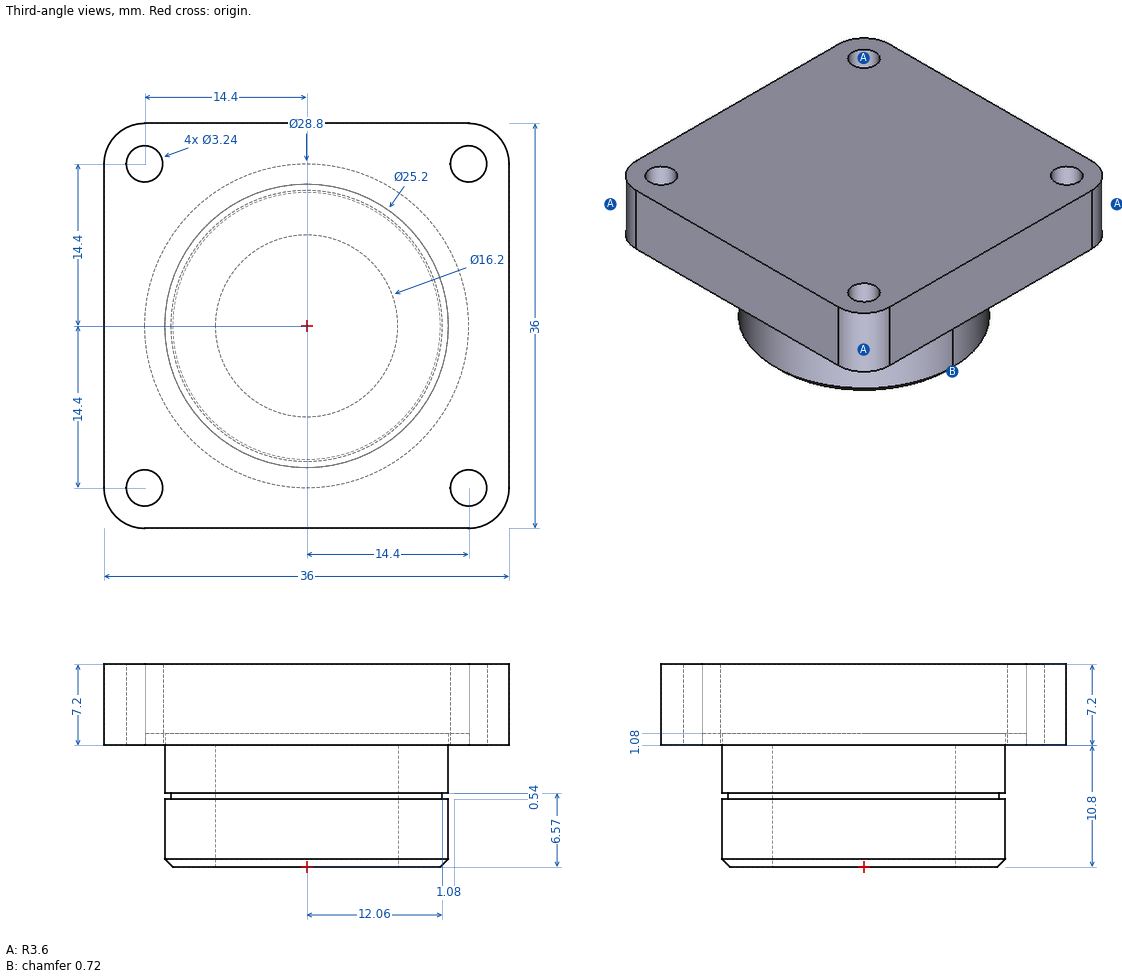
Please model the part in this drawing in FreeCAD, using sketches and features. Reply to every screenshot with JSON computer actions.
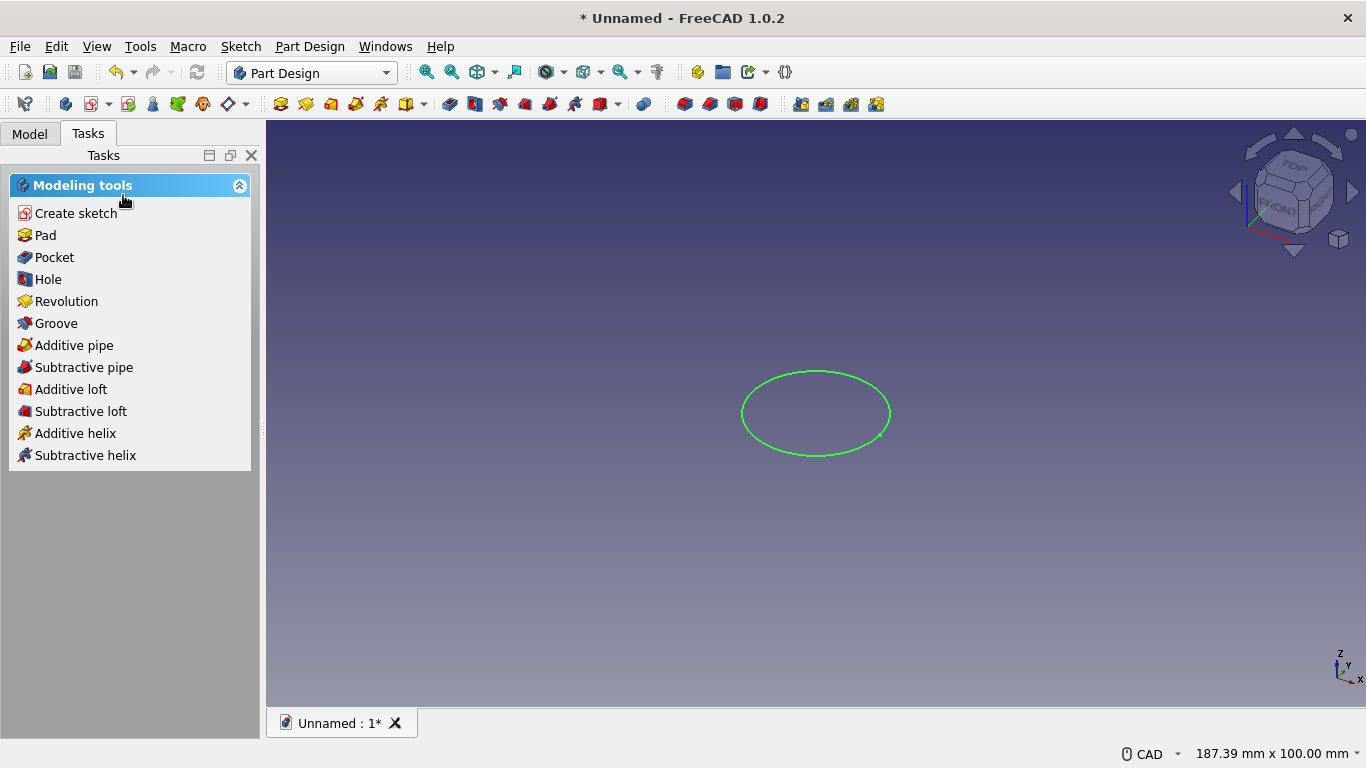
{"action": "left_click", "coordinate": [281, 104]}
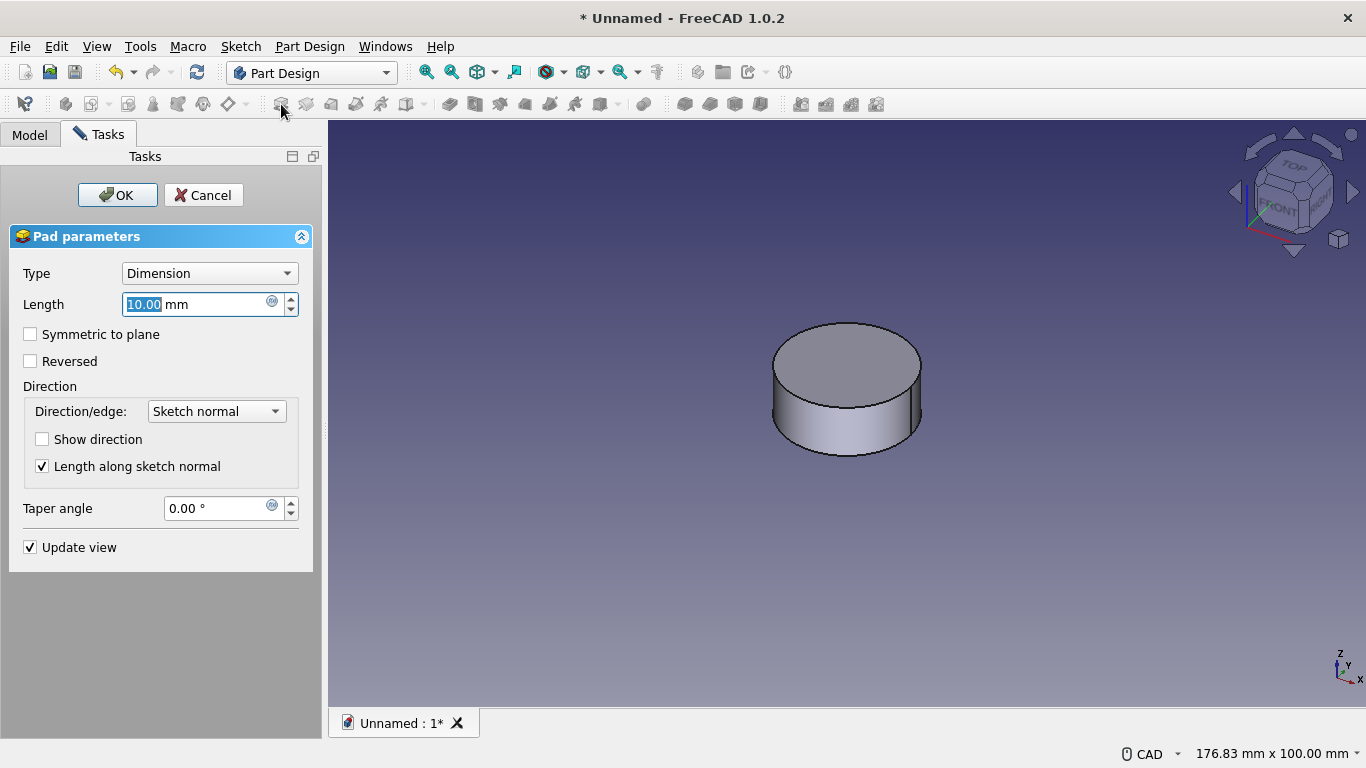
{"action": "type", "text": "10.8"}
{"action": "key", "text": "Tab"}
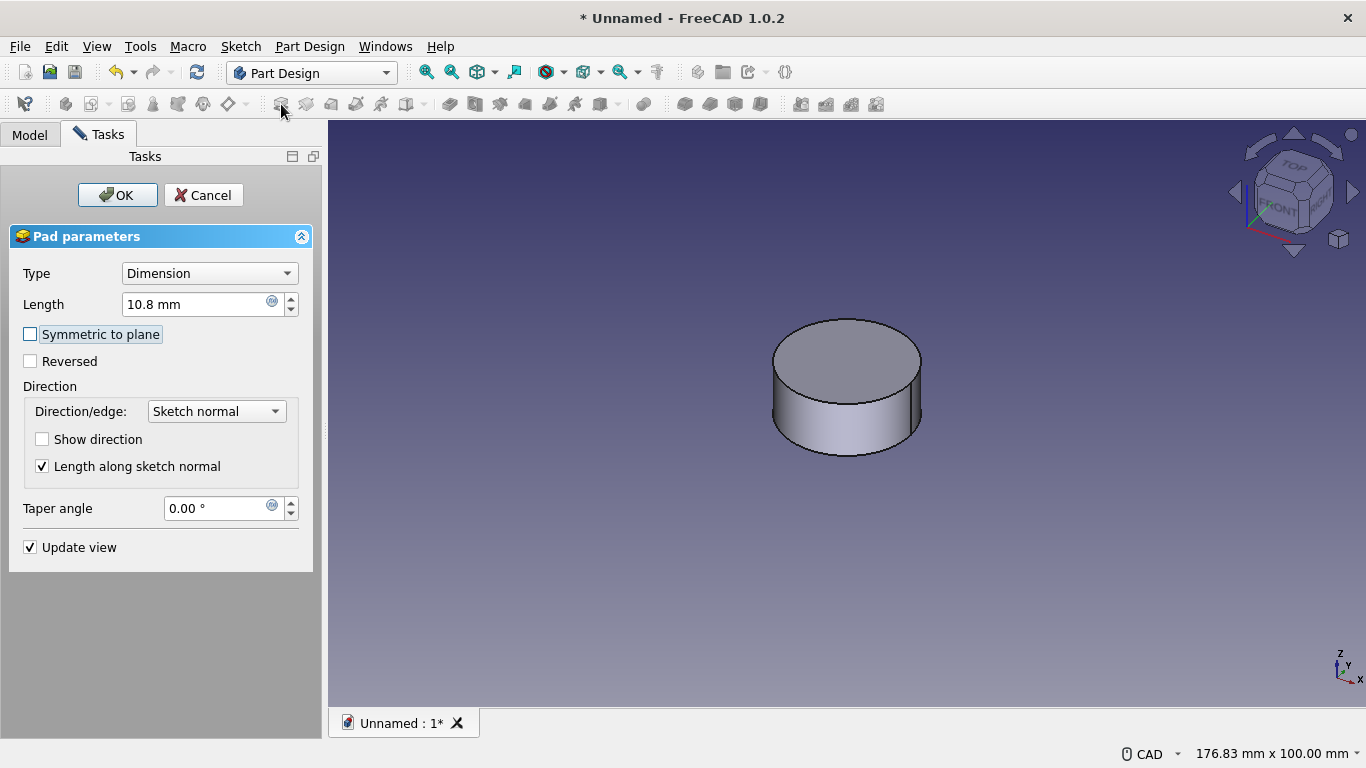
{"action": "left_click", "coordinate": [118, 195]}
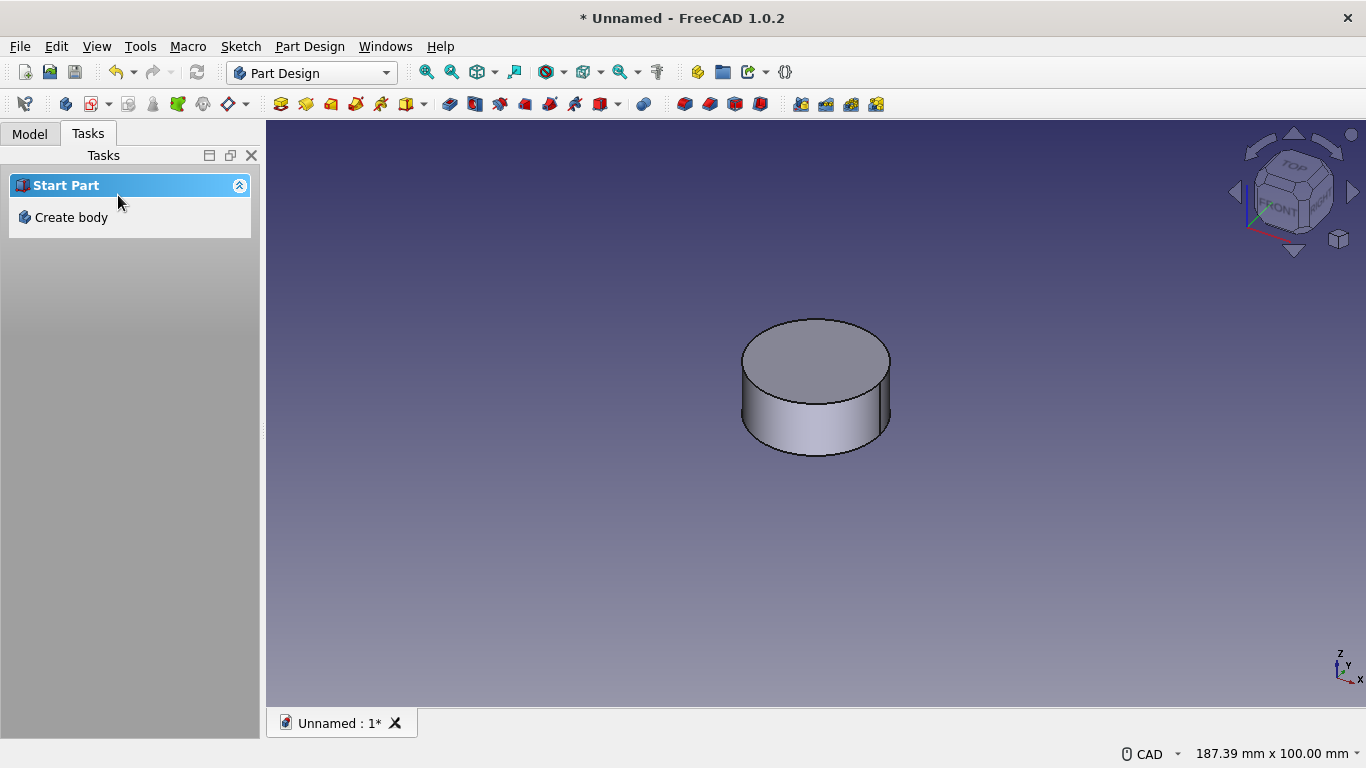
{"action": "left_click", "coordinate": [427, 72]}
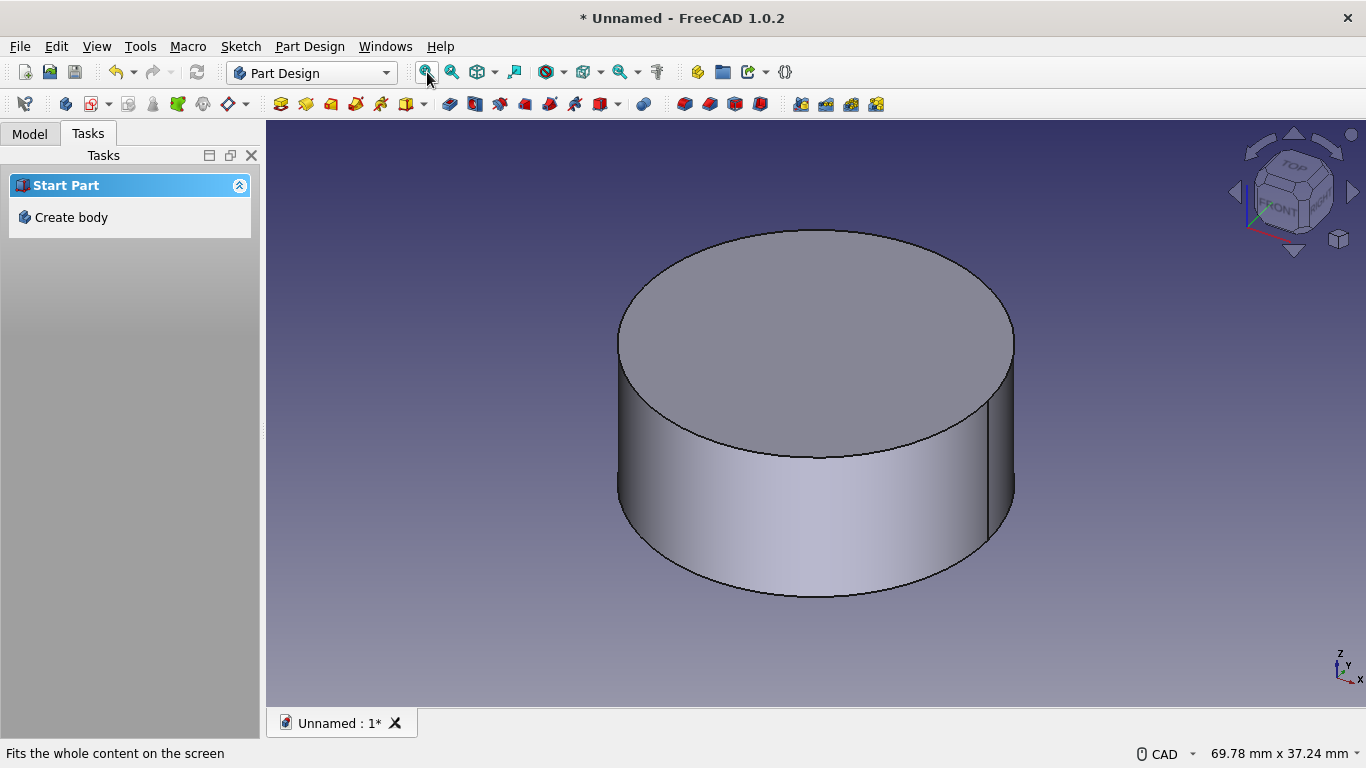
{"action": "left_click", "coordinate": [816, 343]}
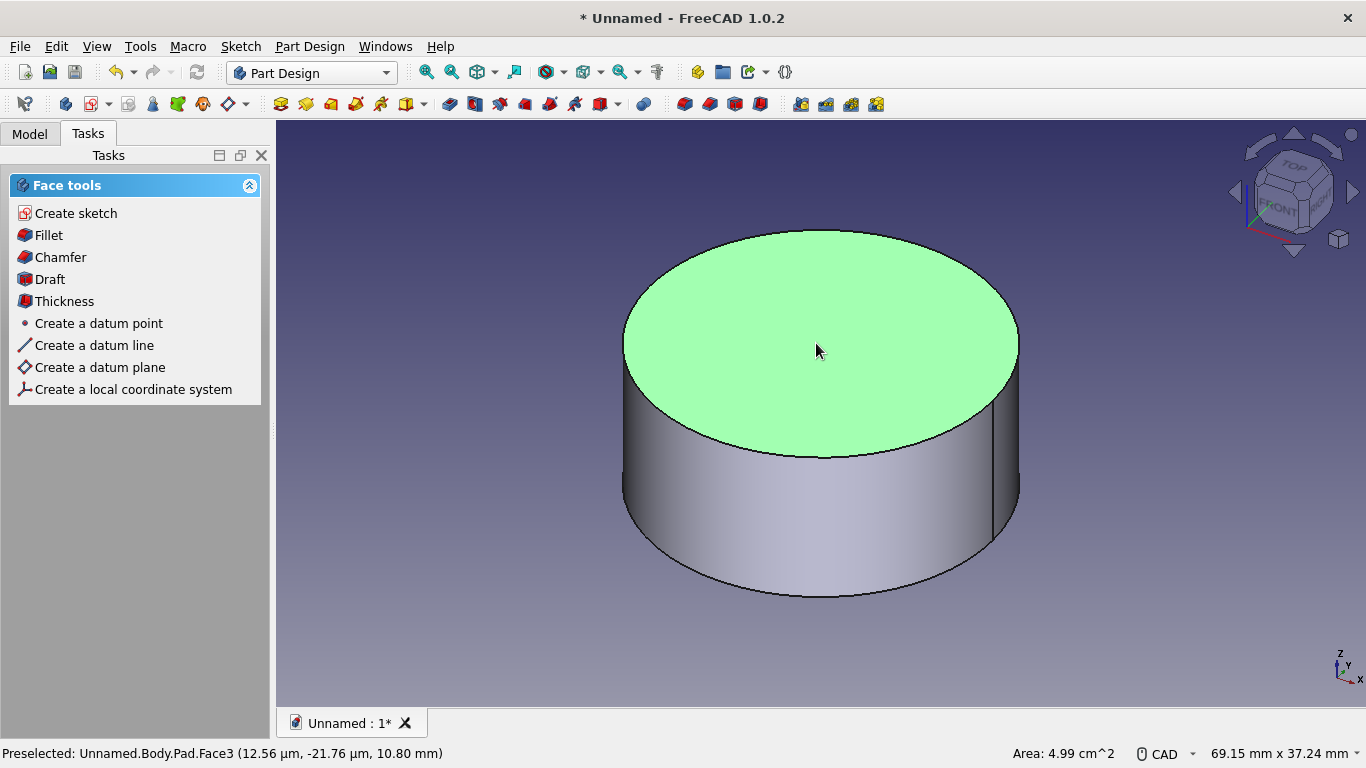
{"action": "left_click", "coordinate": [90, 104]}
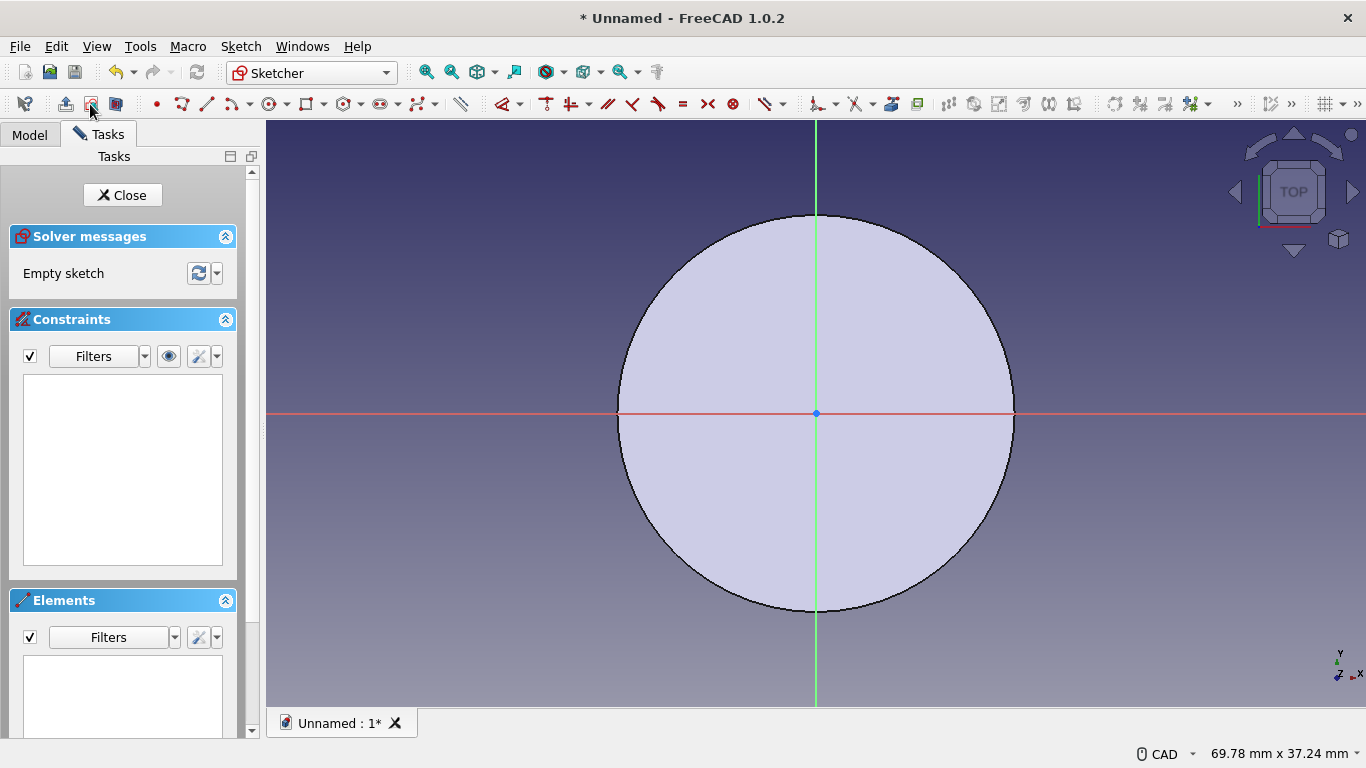
{"action": "scroll", "coordinate": [608, 414], "scroll_direction": "down", "scroll_amount": 2}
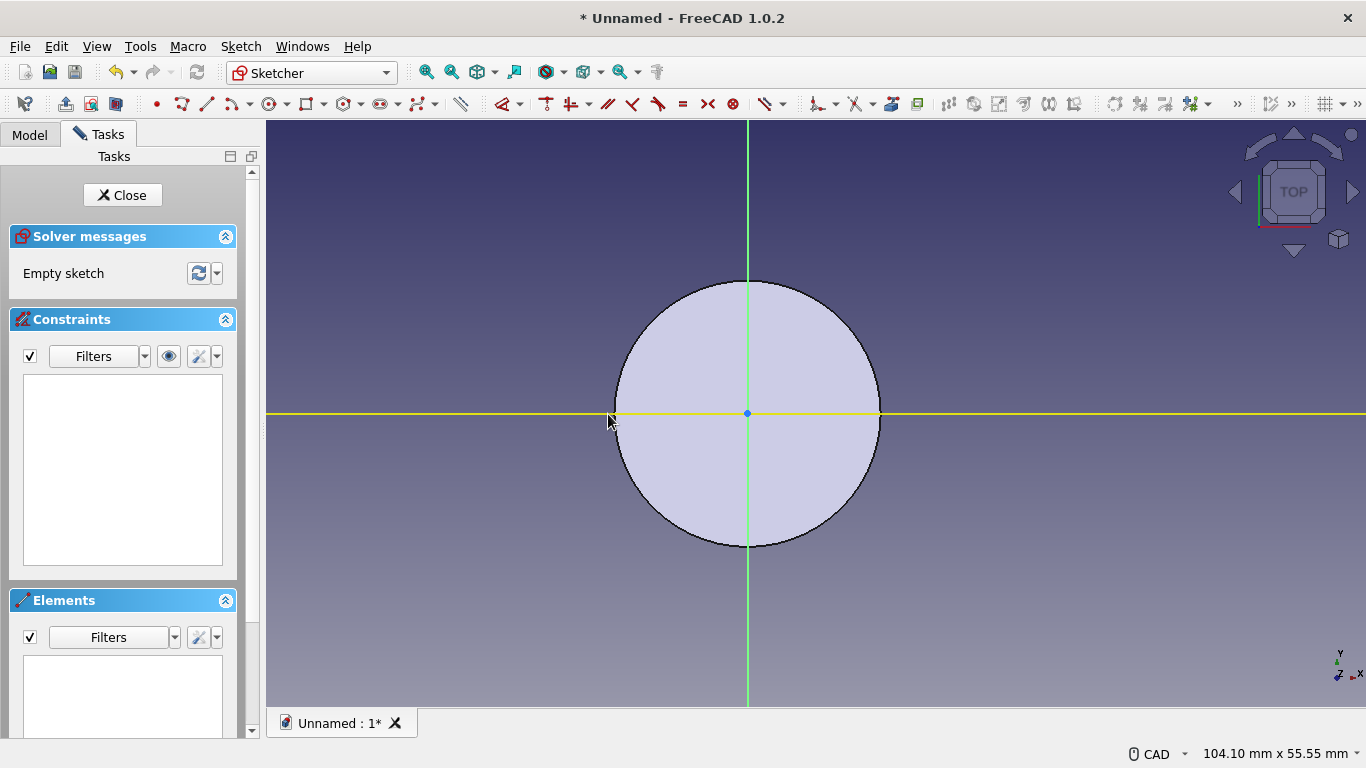
{"action": "left_click", "coordinate": [324, 104]}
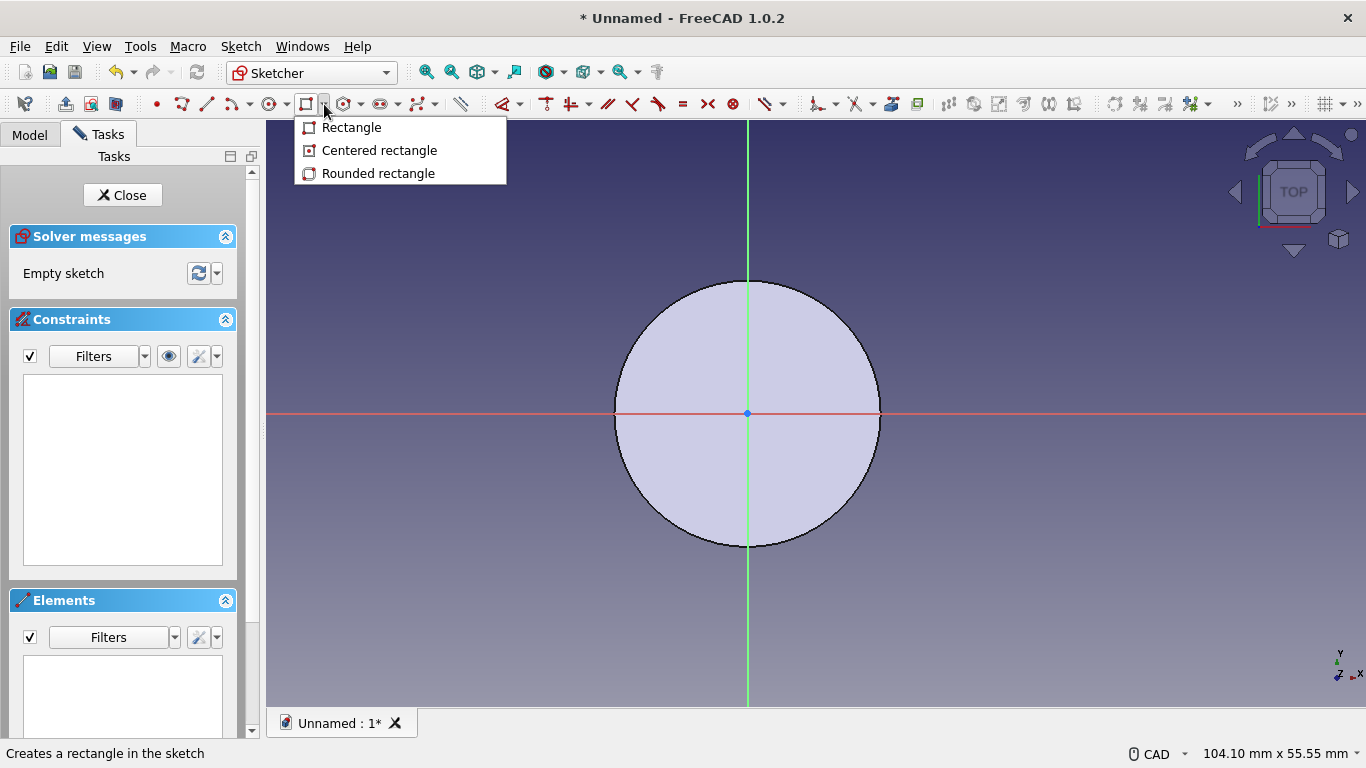
{"action": "left_click", "coordinate": [400, 150]}